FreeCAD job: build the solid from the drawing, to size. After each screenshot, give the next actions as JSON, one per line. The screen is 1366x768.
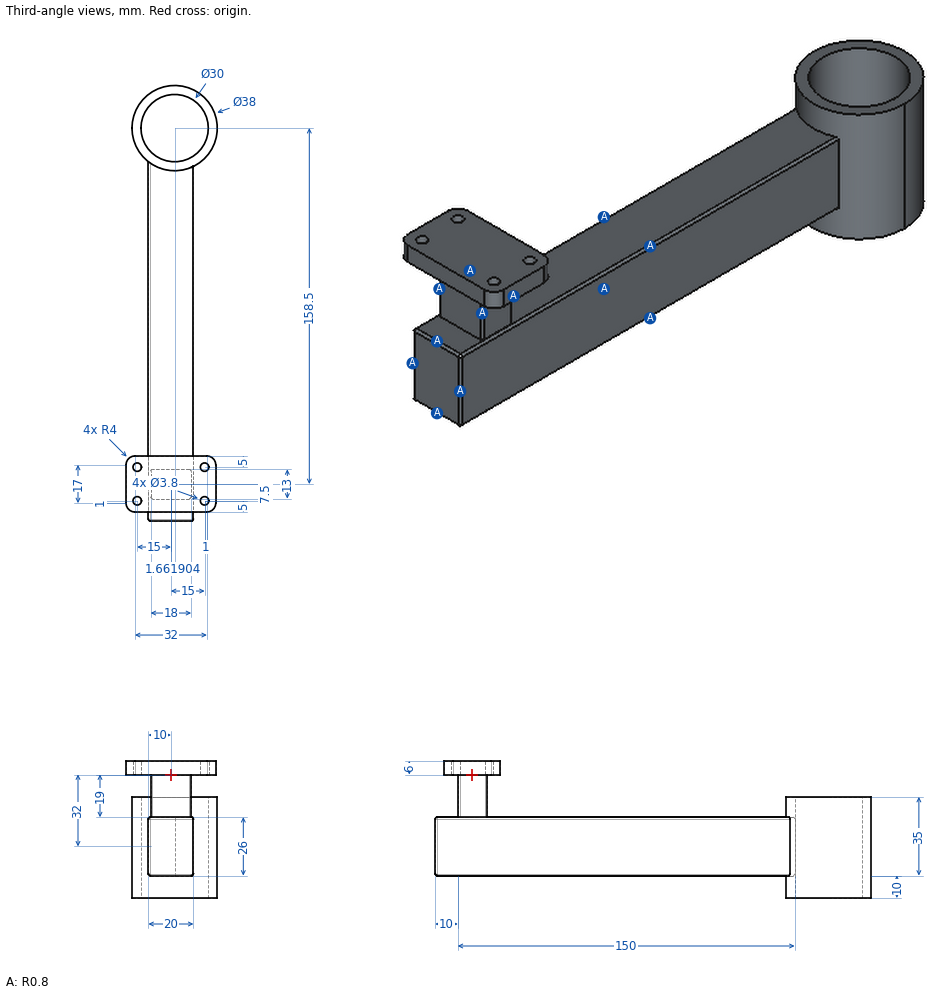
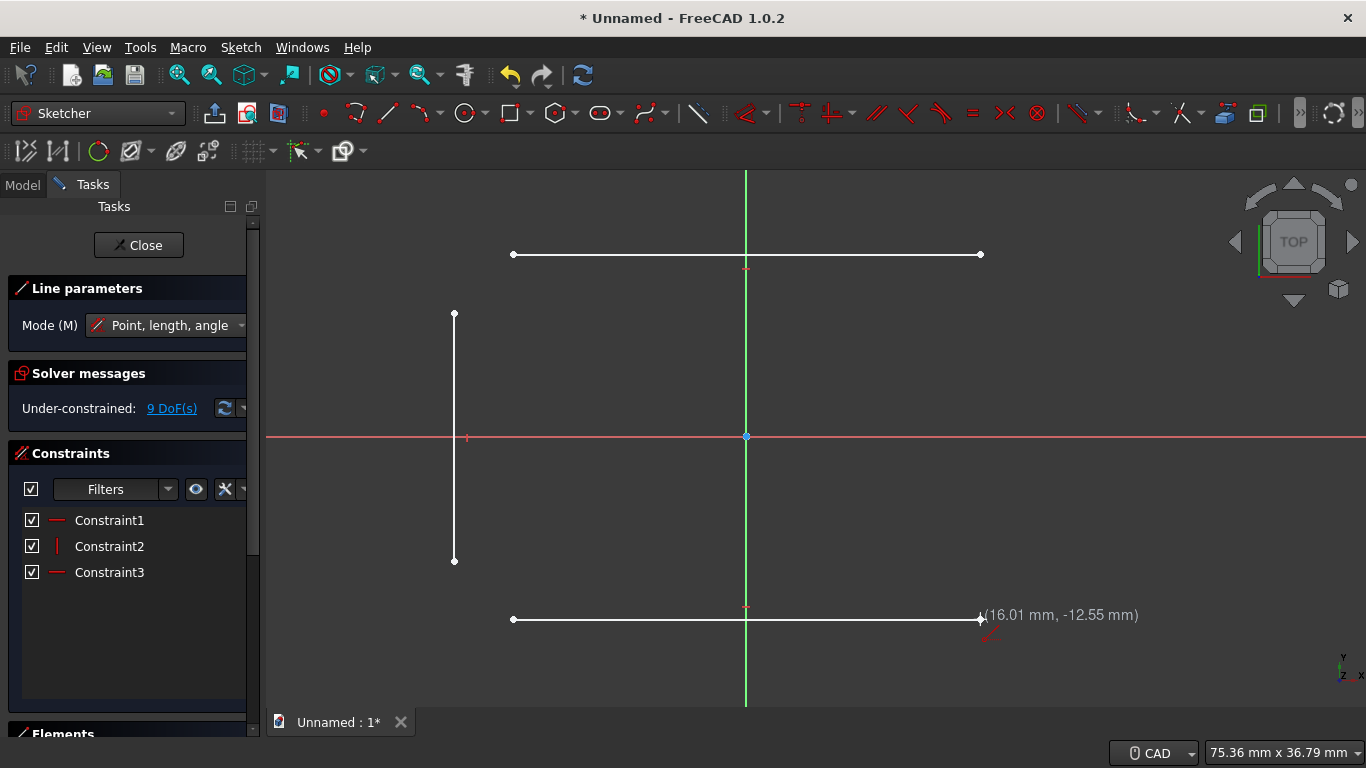
{"action": "left_click", "coordinate": [1038, 561]}
{"action": "left_click", "coordinate": [1038, 313]}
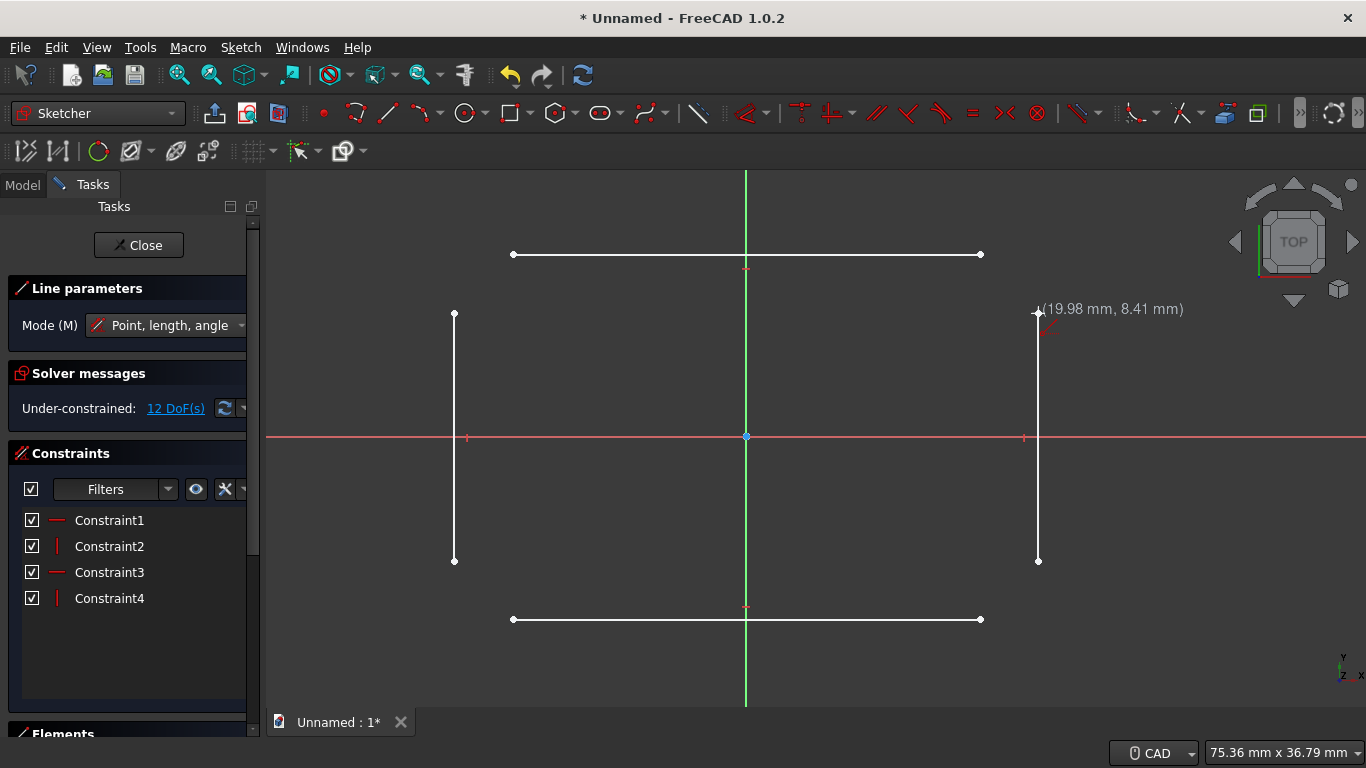
{"action": "left_click", "coordinate": [420, 114]}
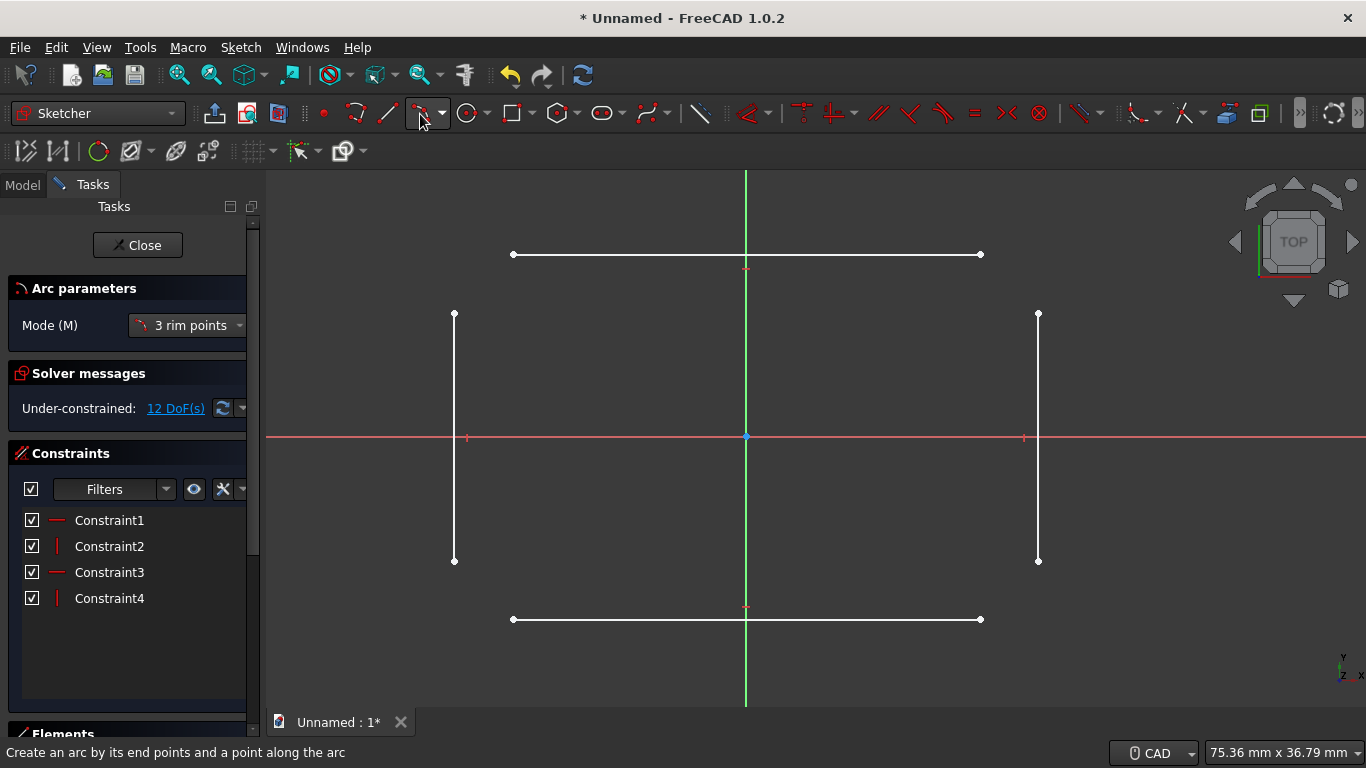
{"action": "left_click", "coordinate": [513, 255]}
{"action": "left_click", "coordinate": [454, 314]}
{"action": "left_click", "coordinate": [472, 271]}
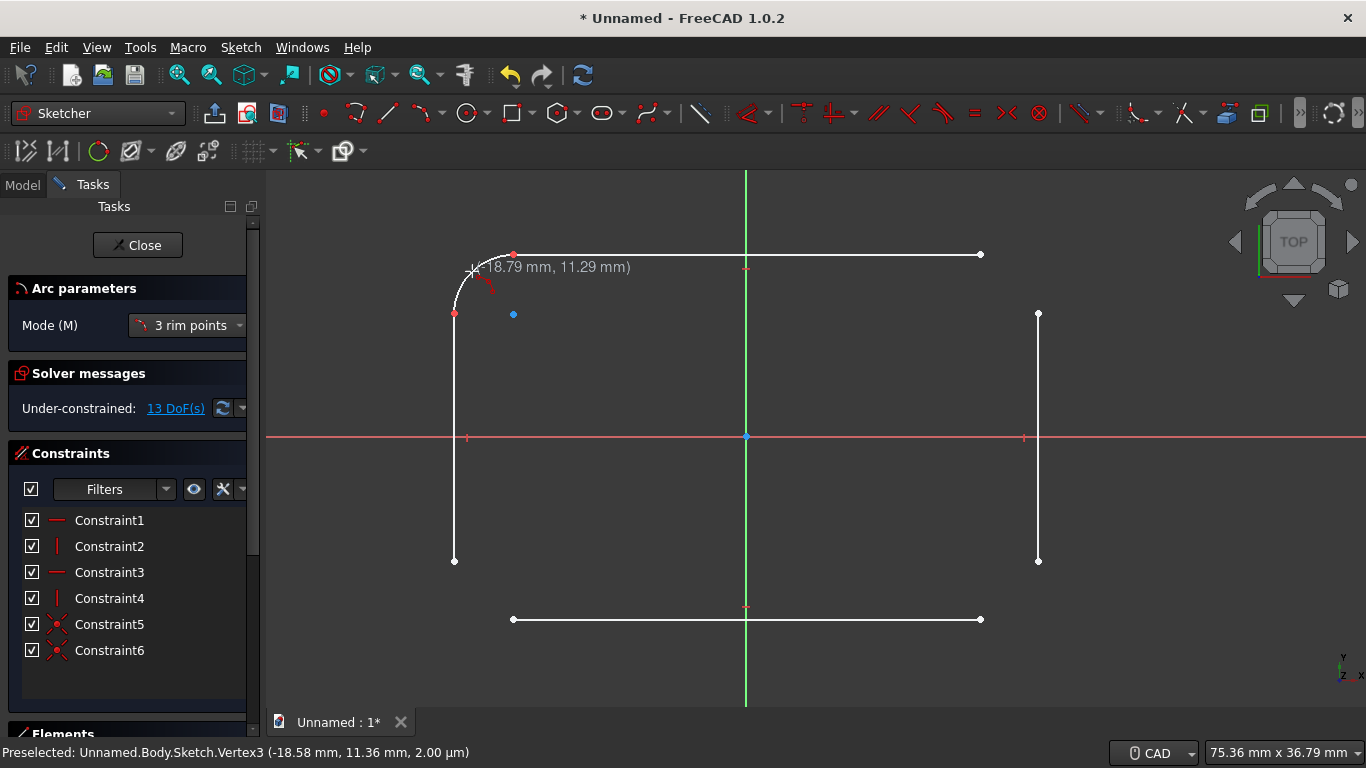
{"action": "left_click", "coordinate": [454, 562]}
{"action": "left_click", "coordinate": [513, 620]}
{"action": "left_click", "coordinate": [472, 602]}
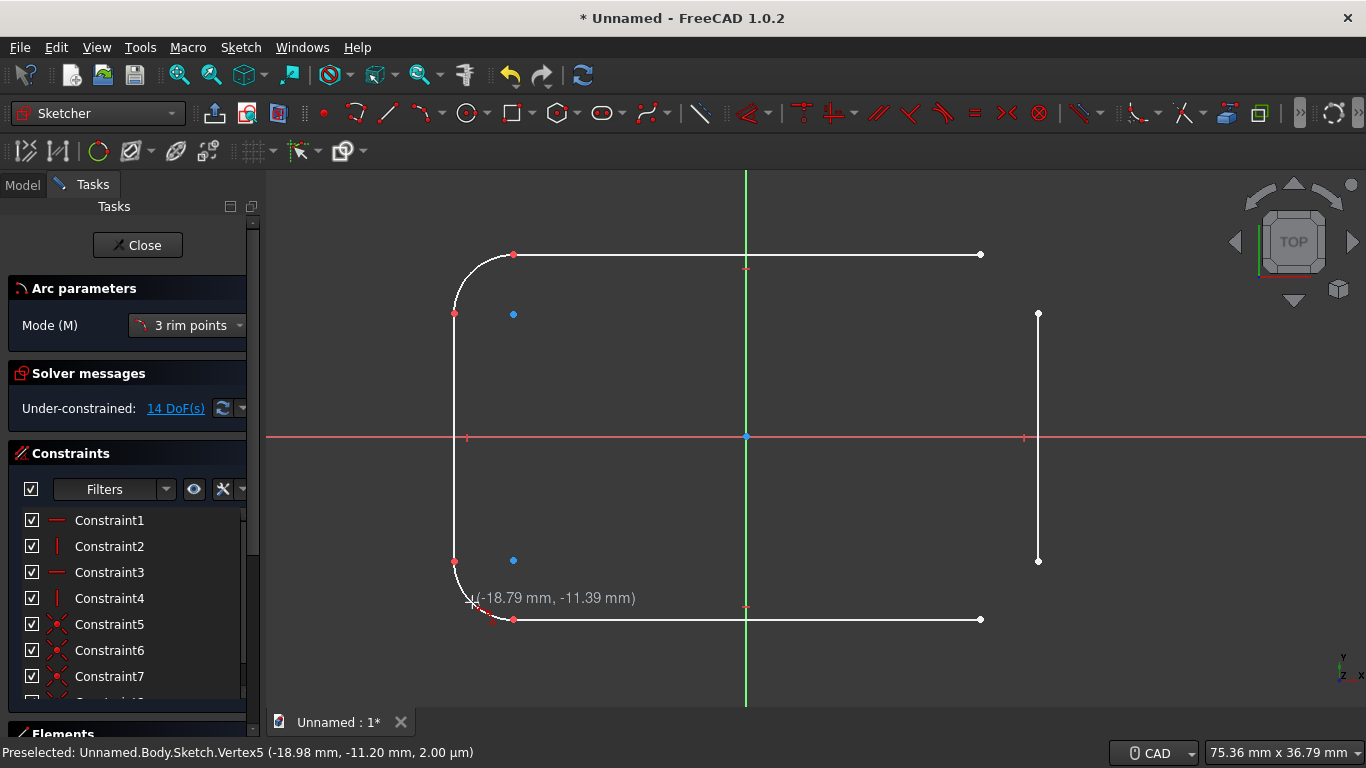
{"action": "left_click", "coordinate": [980, 620]}
{"action": "left_click", "coordinate": [1038, 562]}
{"action": "left_click", "coordinate": [1021, 602]}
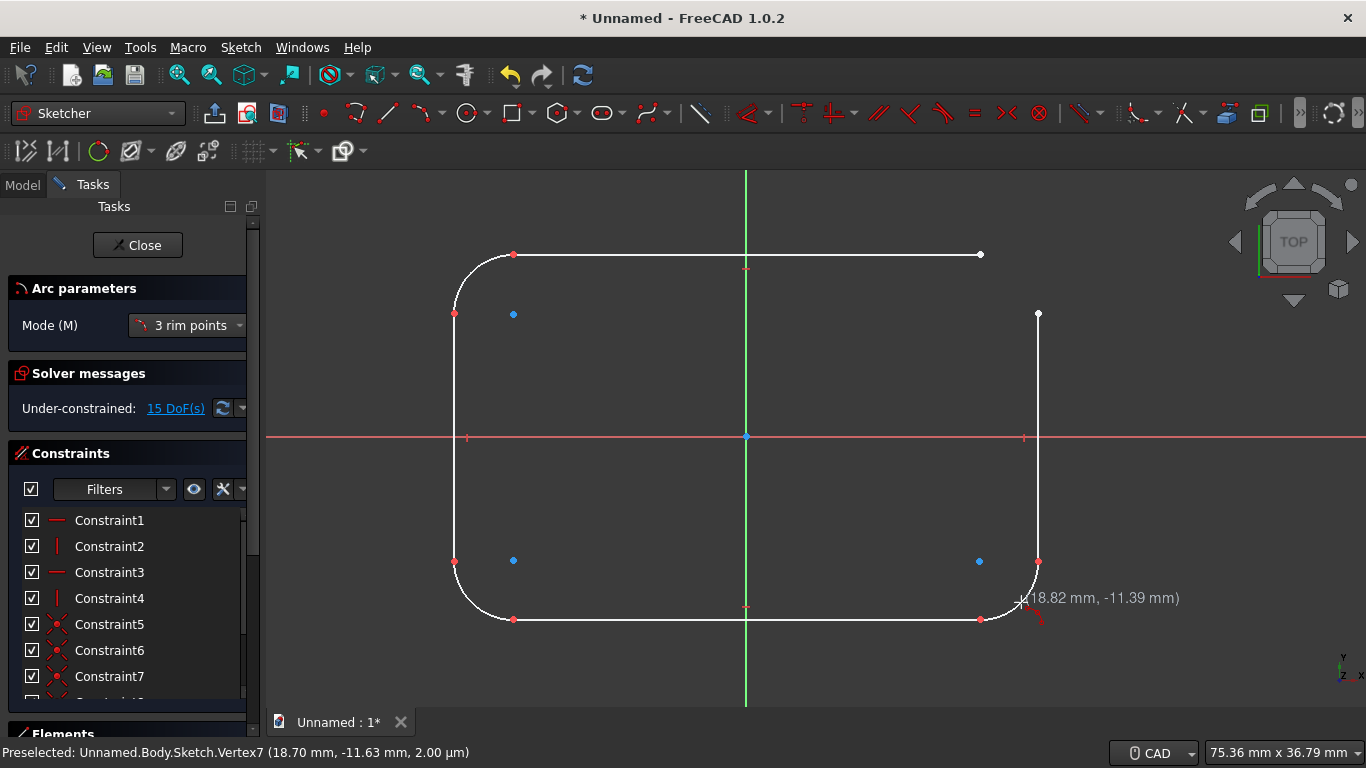
{"action": "left_click", "coordinate": [1038, 314]}
{"action": "left_click", "coordinate": [980, 255]}
{"action": "left_click", "coordinate": [1021, 271]}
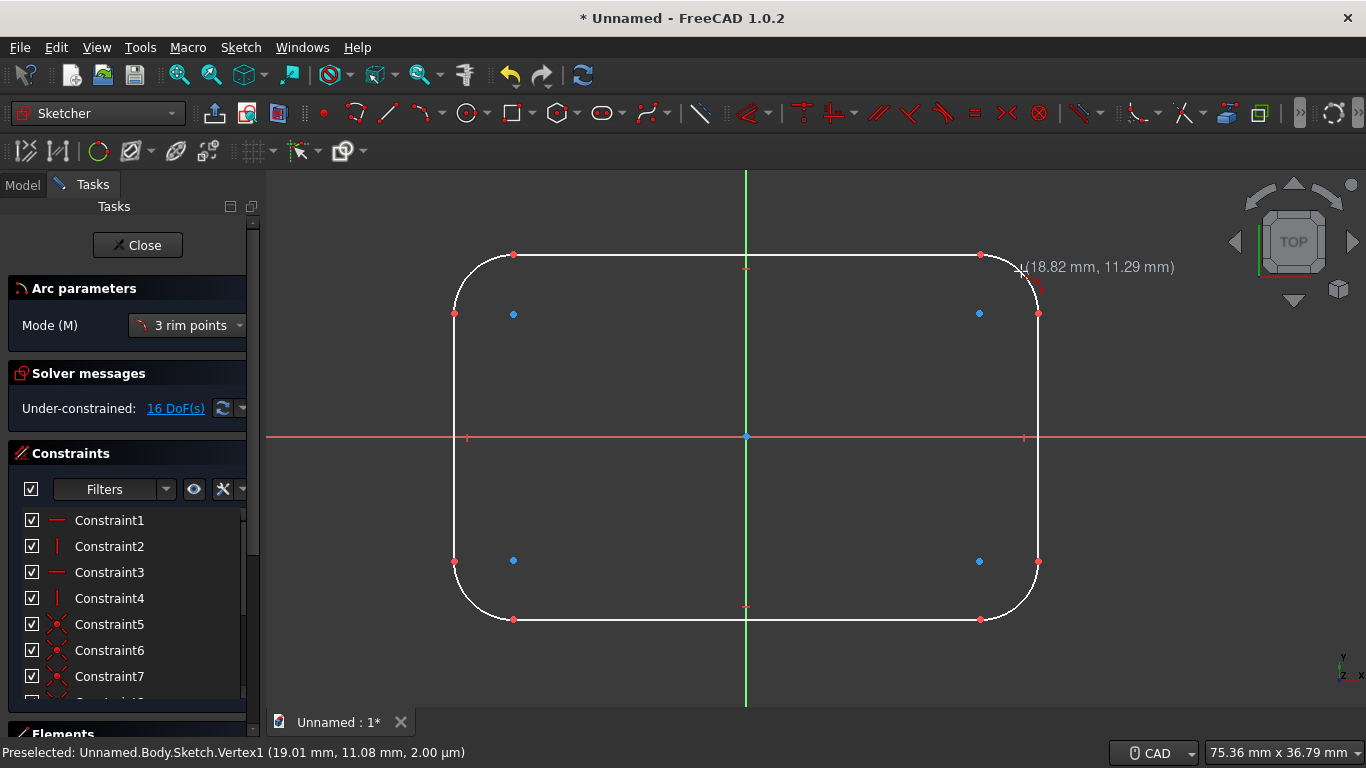
{"action": "left_click", "coordinate": [468, 114]}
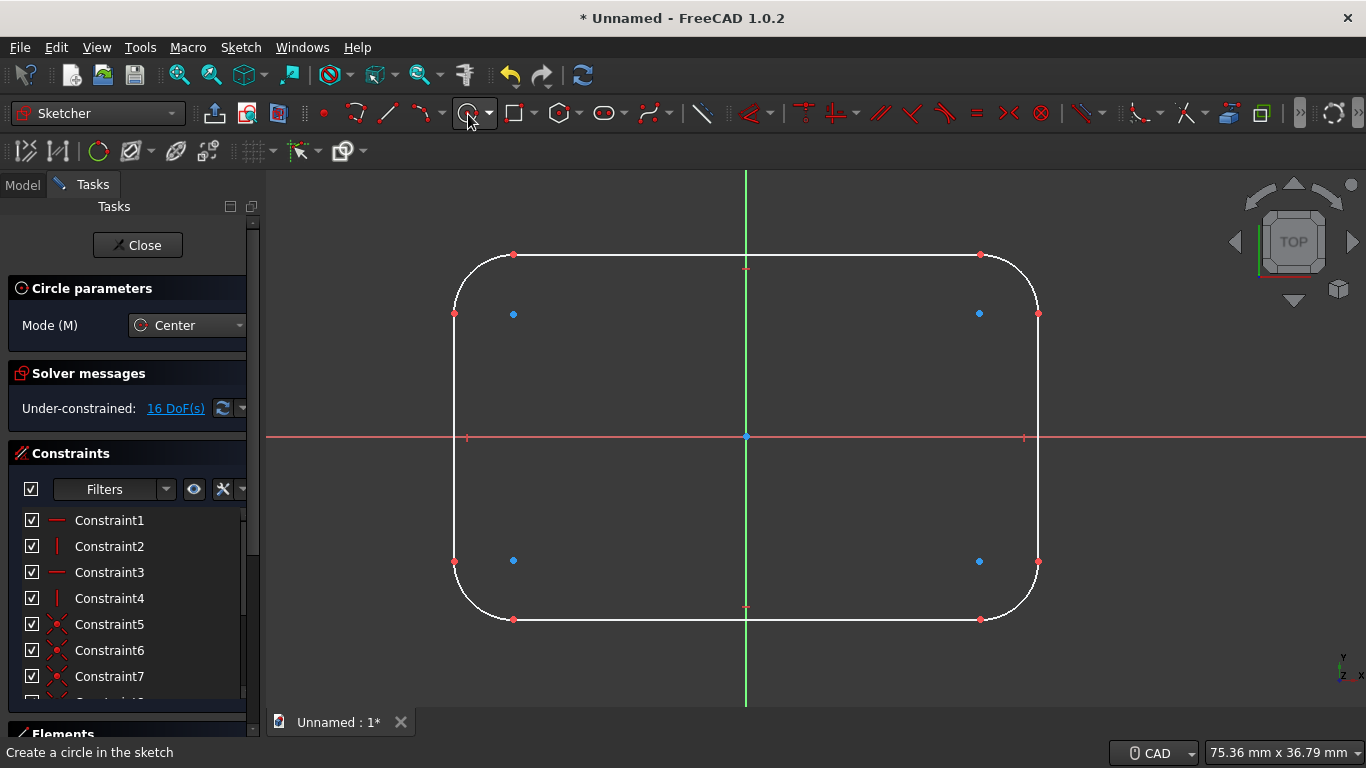
{"action": "left_click", "coordinate": [965, 546]}
{"action": "mouse_move", "coordinate": [985, 527]}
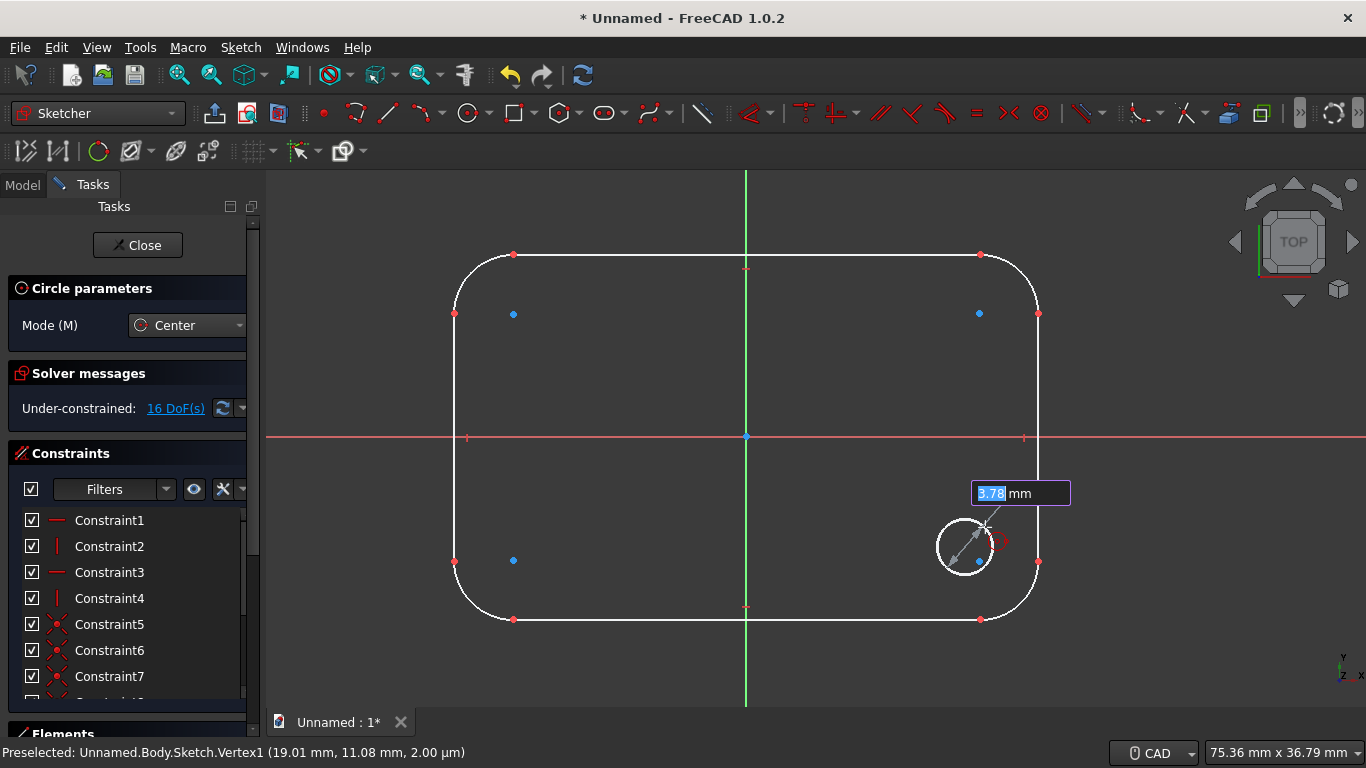
{"action": "type", "text": "3.8"}
{"action": "key", "text": "Return"}